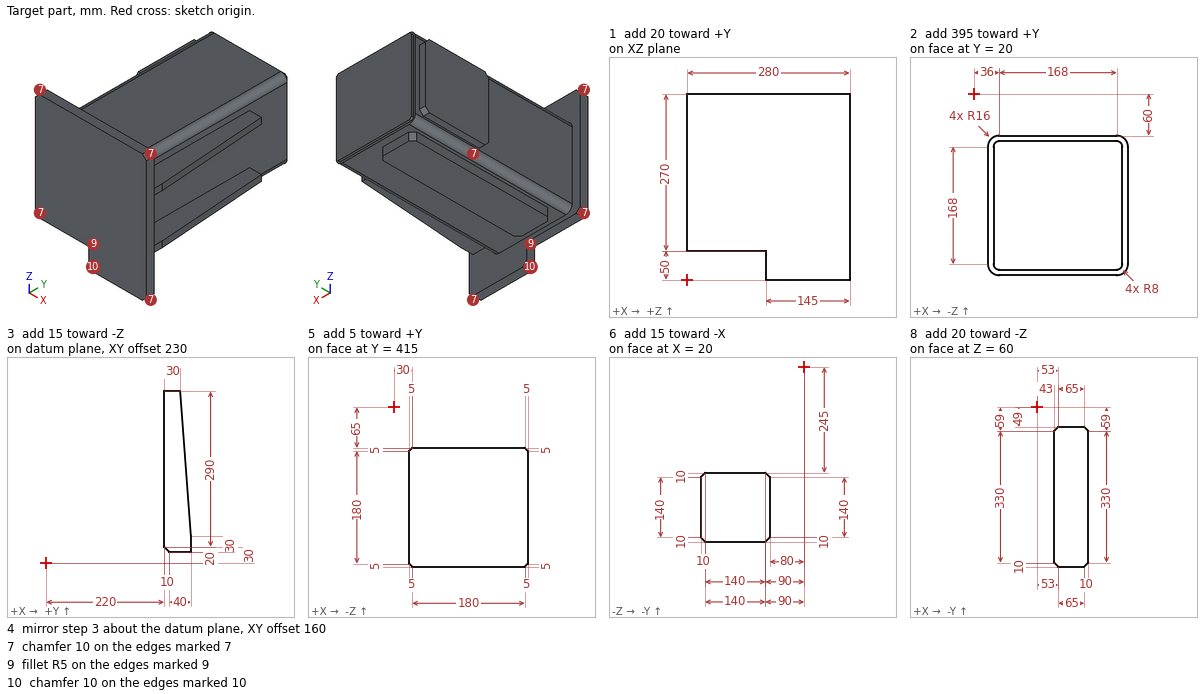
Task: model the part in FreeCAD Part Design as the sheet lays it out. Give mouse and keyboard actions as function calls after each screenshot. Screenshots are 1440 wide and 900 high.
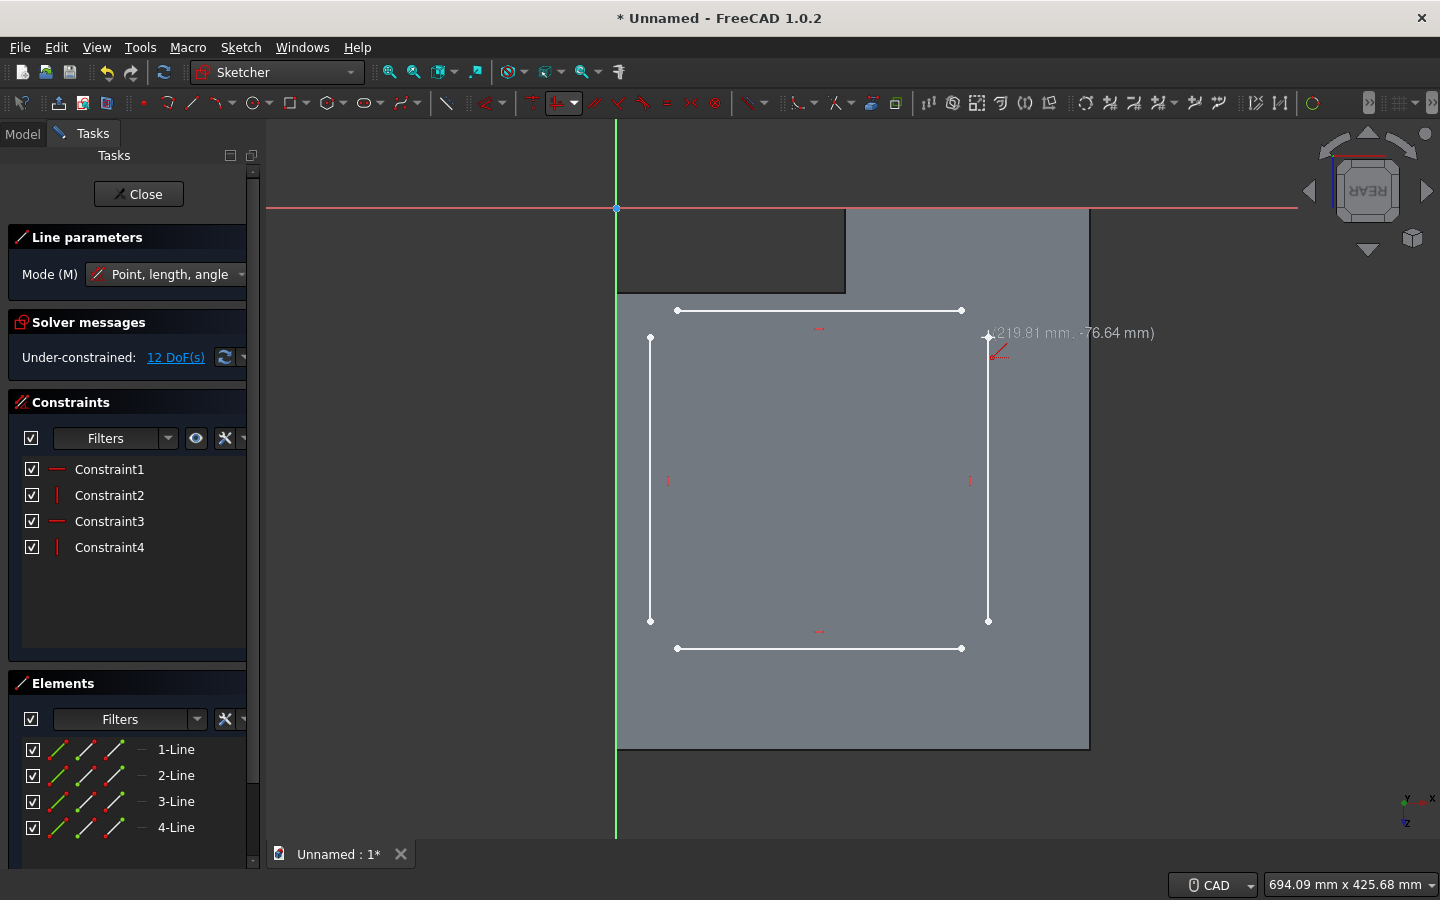
click(216, 104)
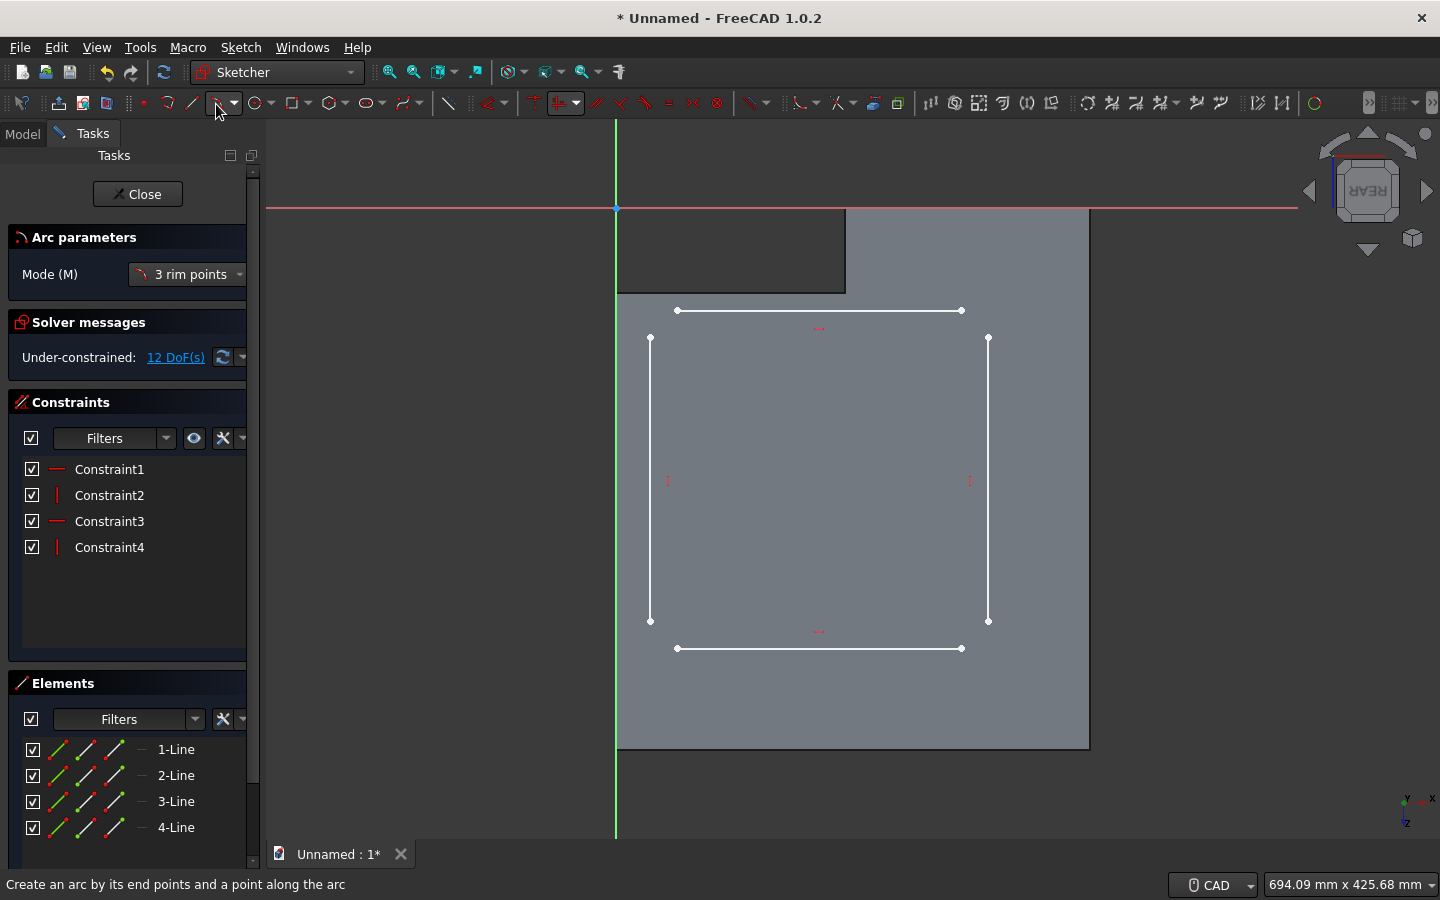
click(677, 311)
click(650, 338)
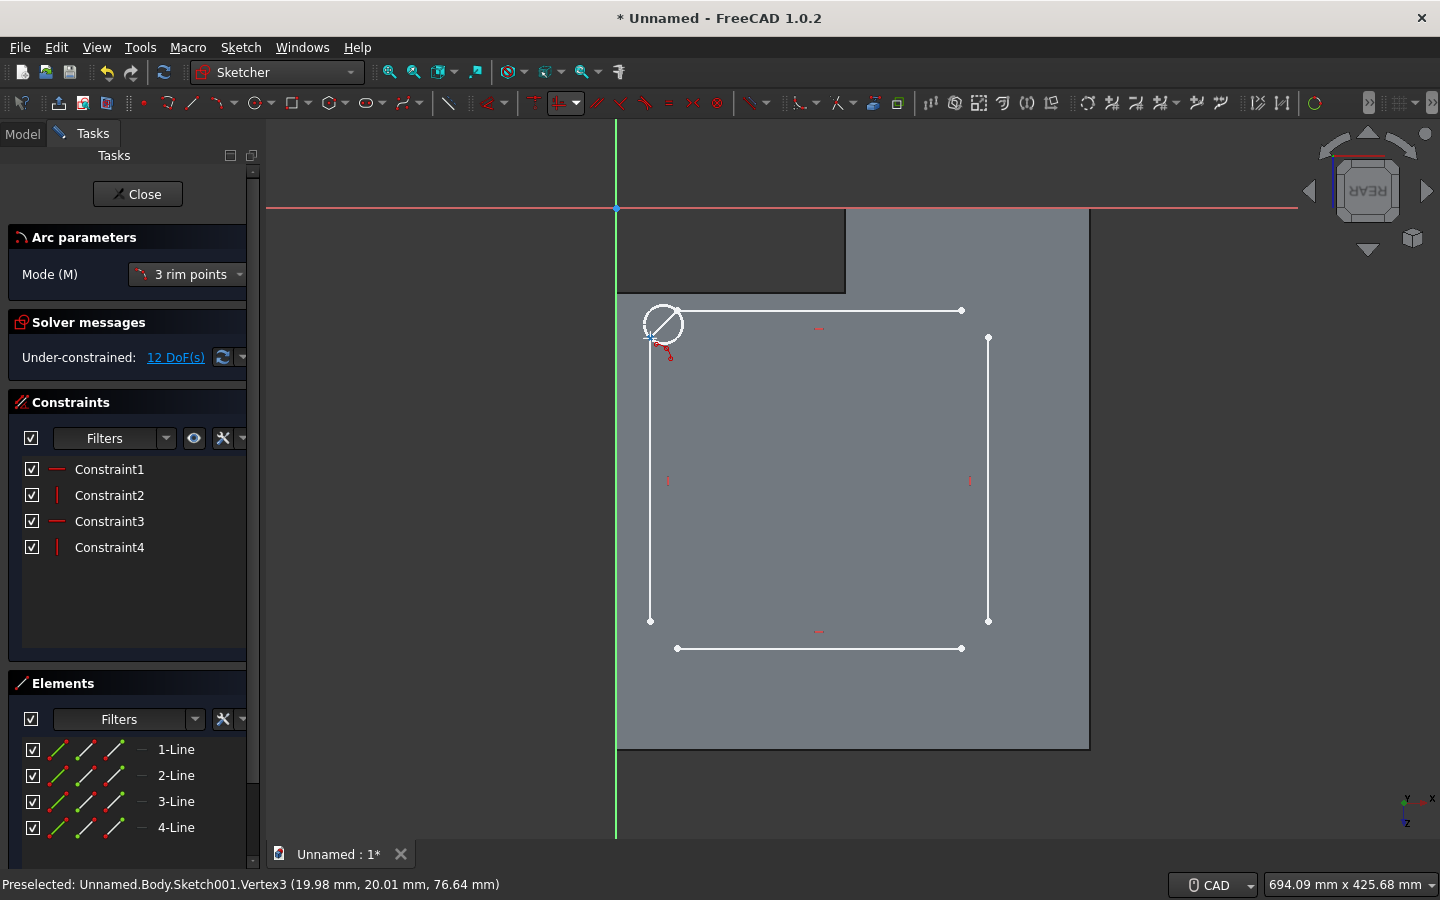
scroll(658, 318, up, 4)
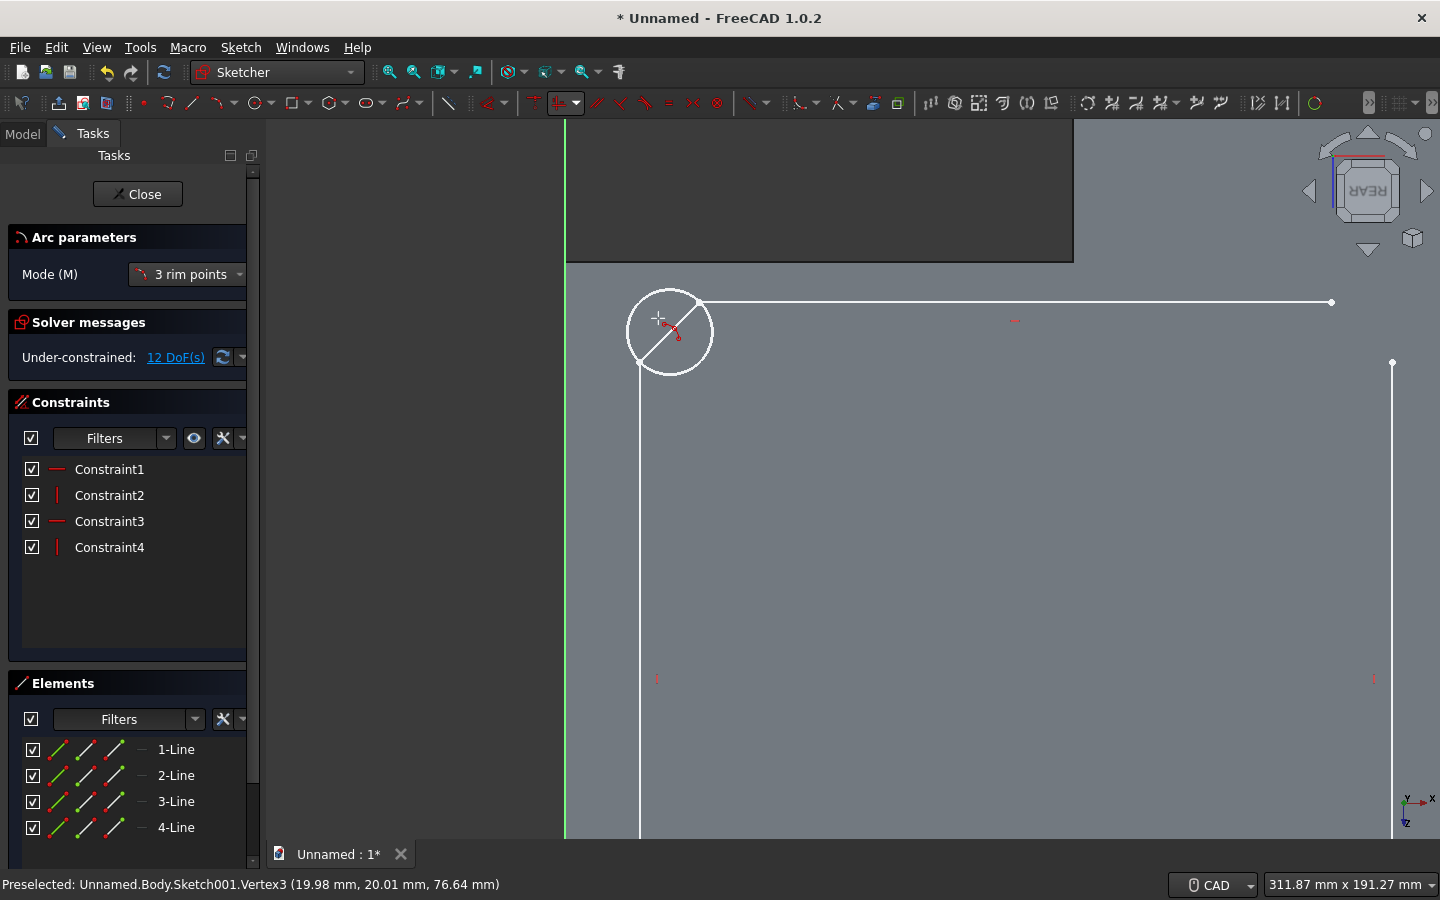
click(657, 317)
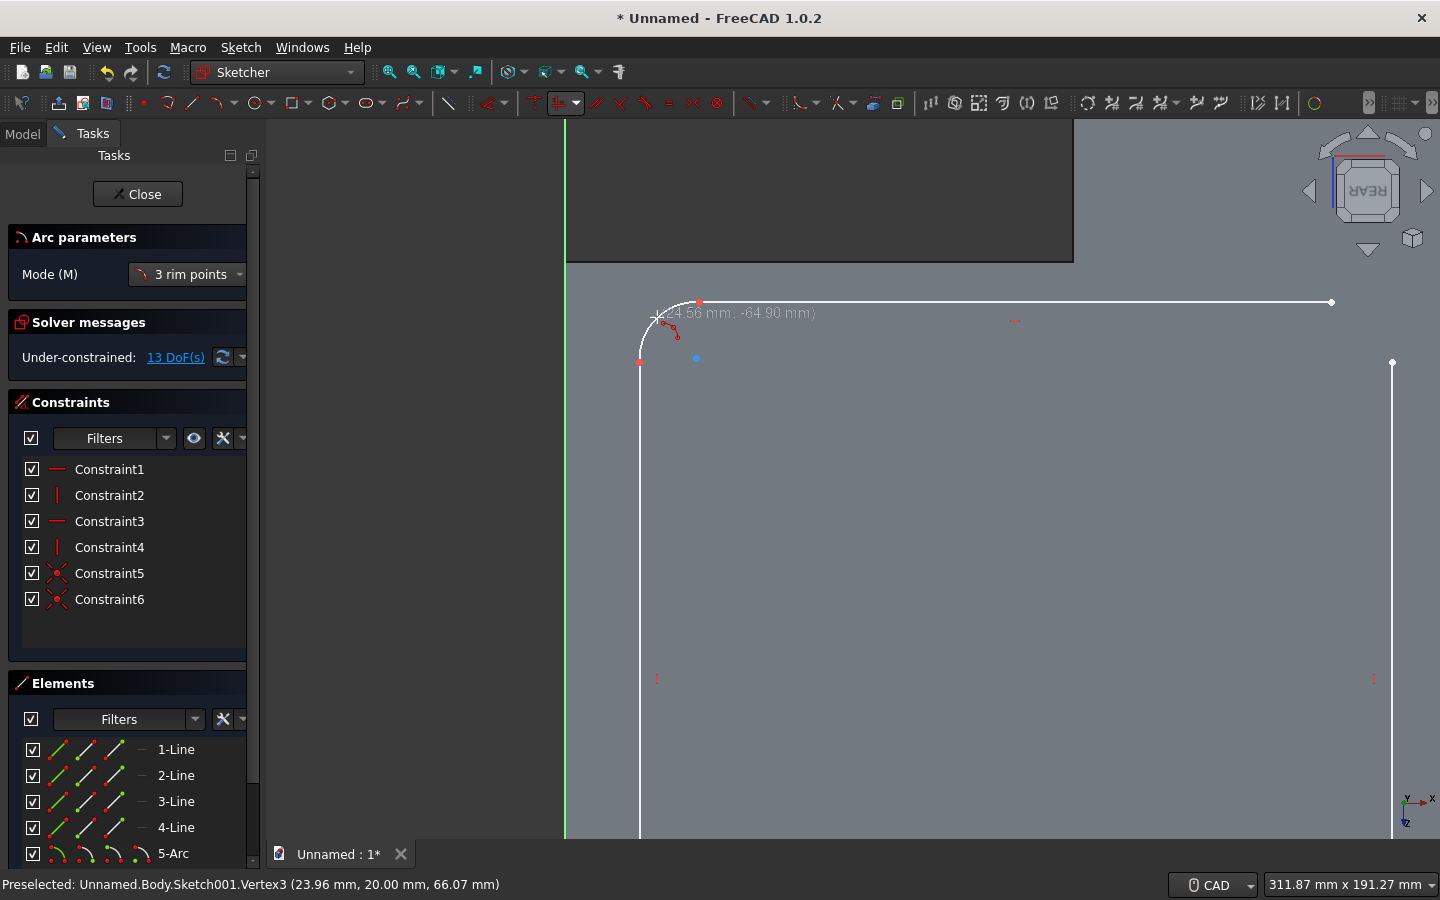
scroll(626, 410, down, 4)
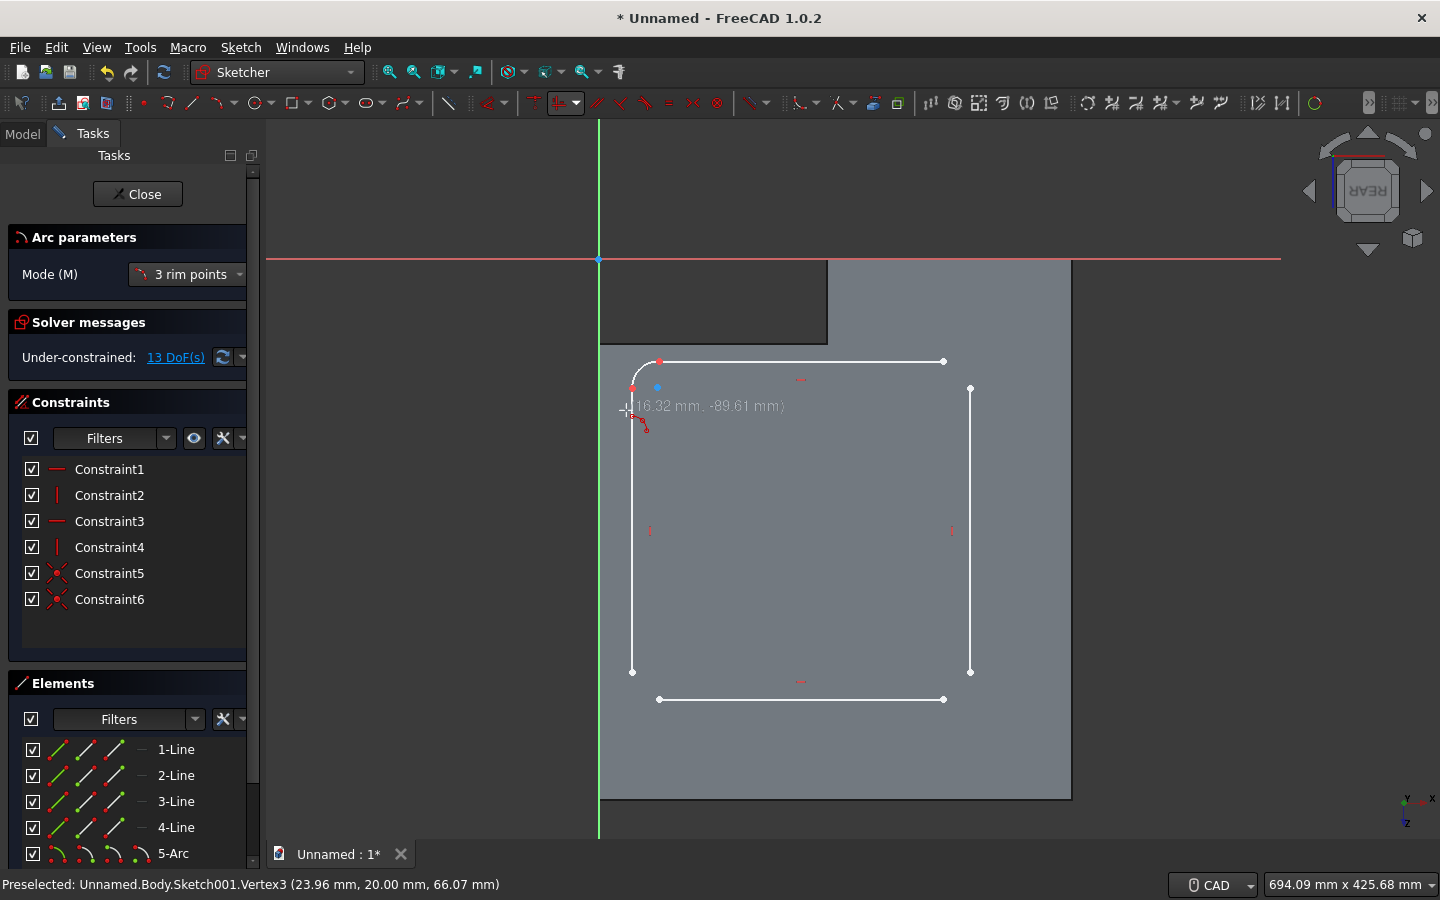
click(632, 673)
click(659, 700)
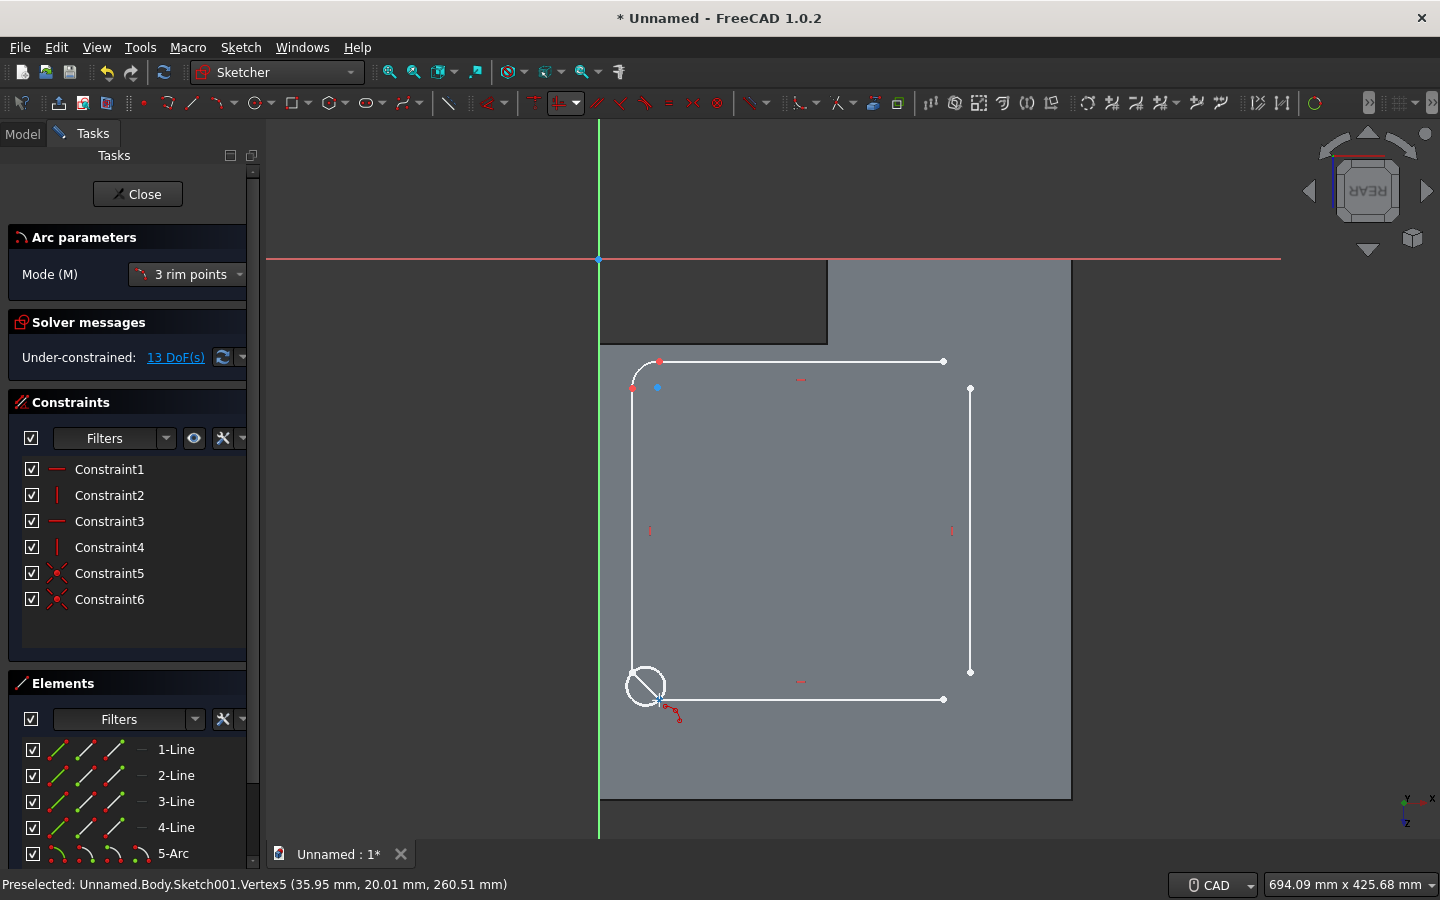
scroll(640, 691, up, 4)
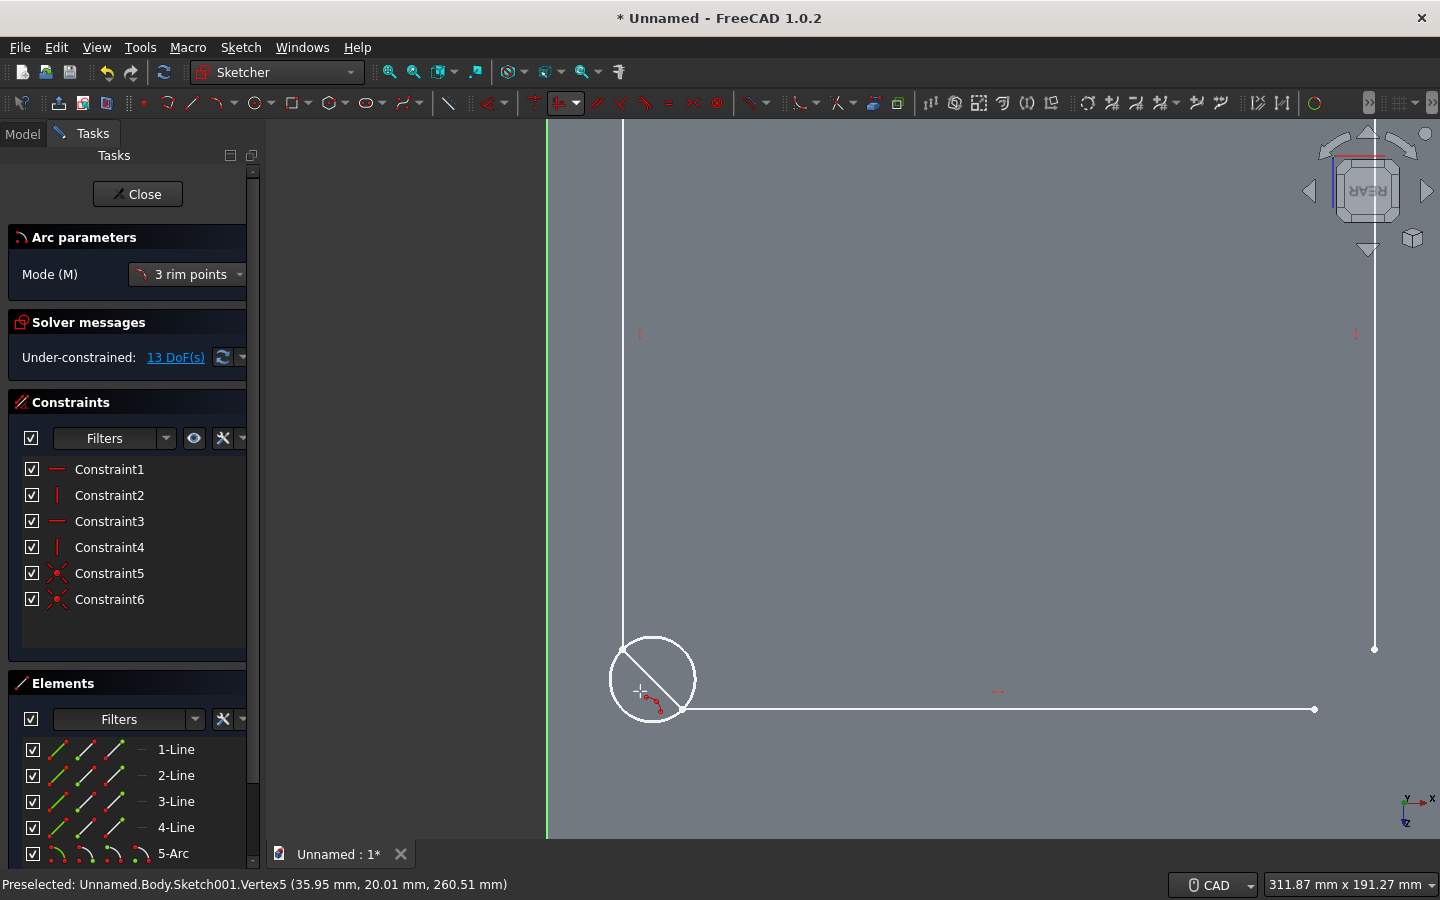
click(640, 690)